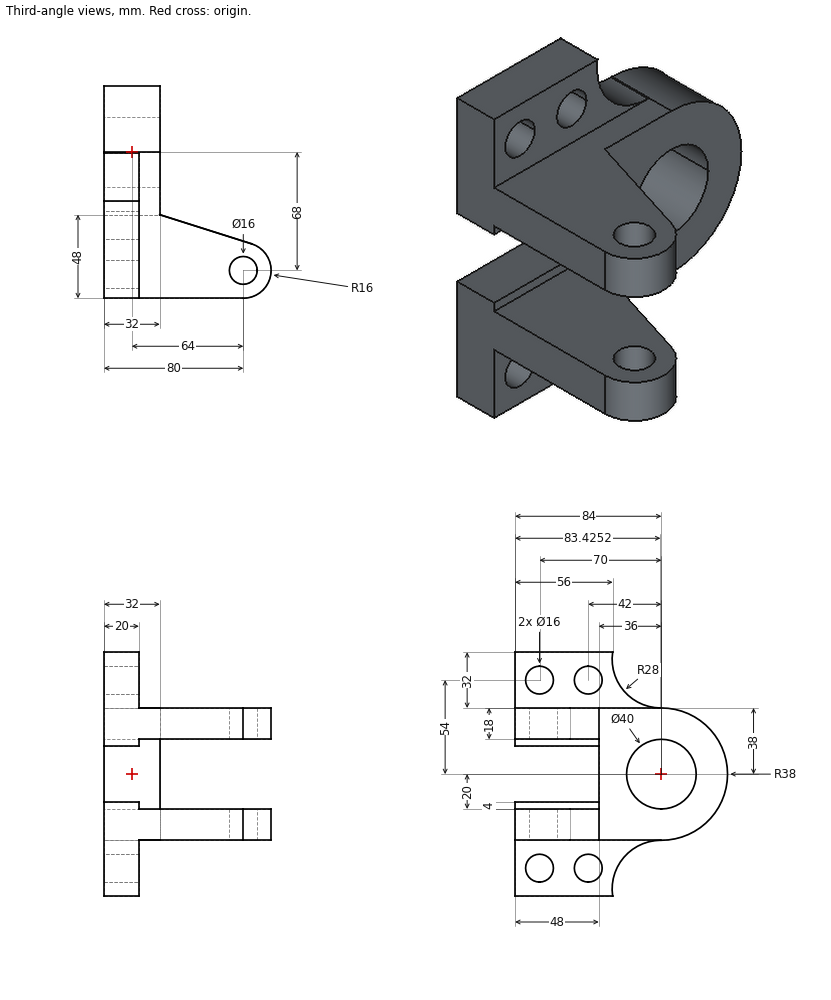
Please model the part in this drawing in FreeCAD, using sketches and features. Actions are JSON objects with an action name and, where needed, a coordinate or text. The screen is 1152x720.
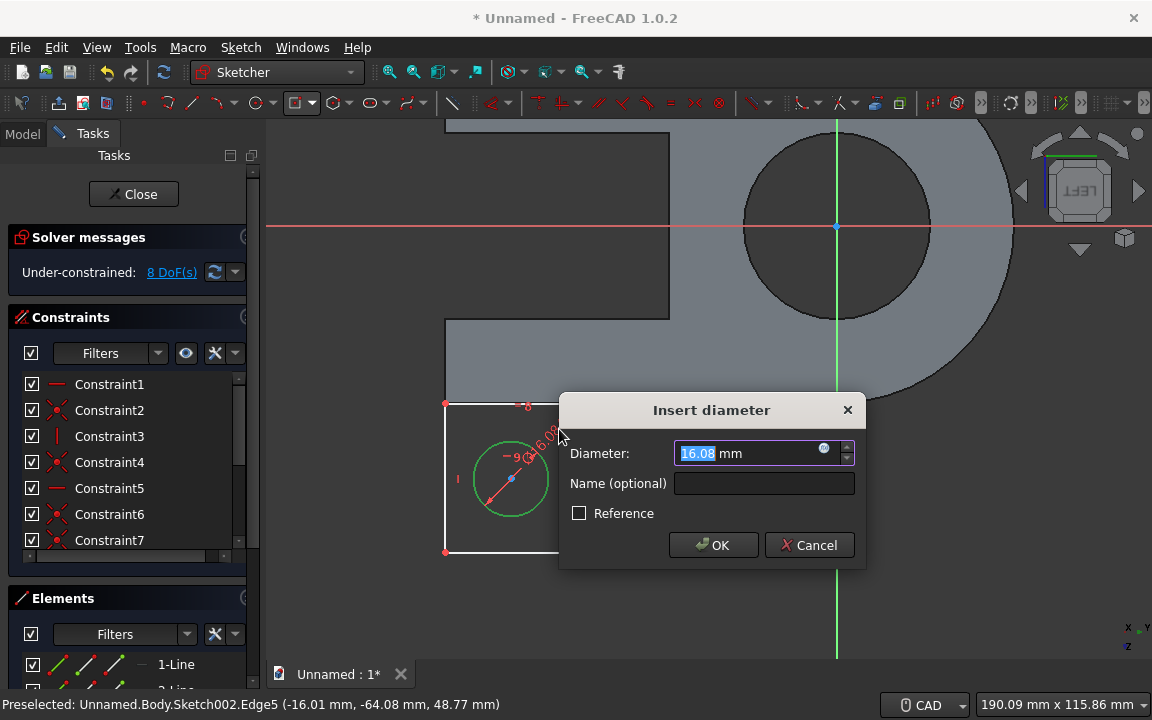
{"action": "type", "text": "16"}
{"action": "key", "text": "Return"}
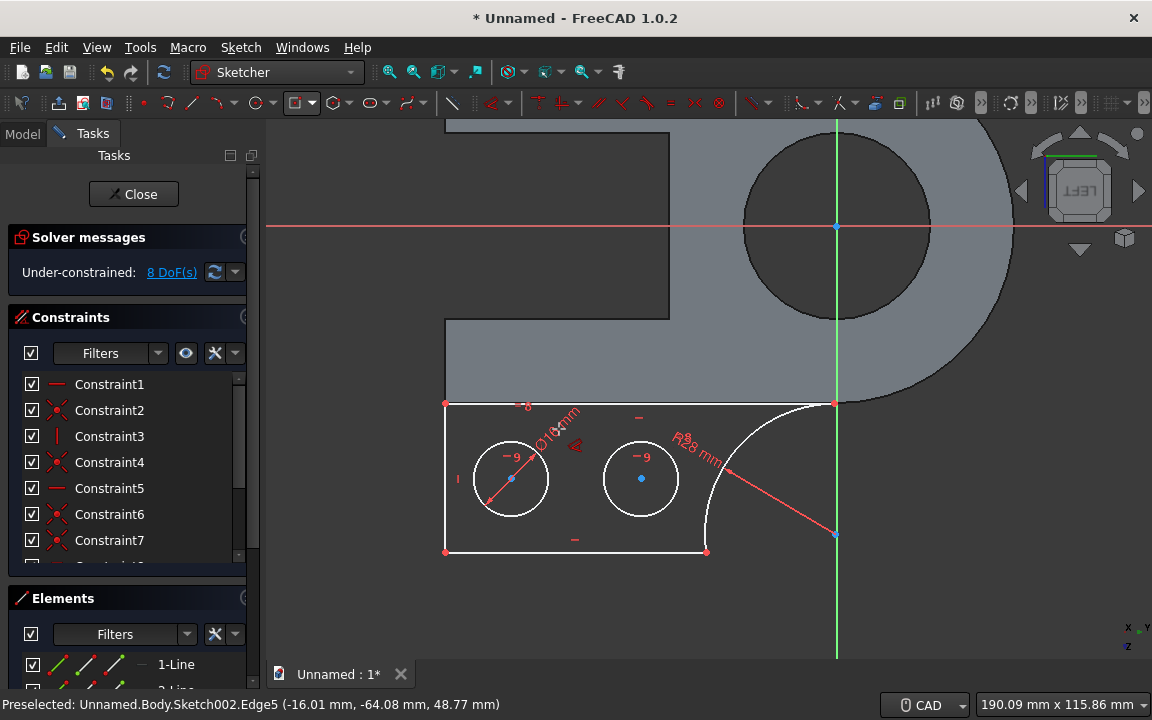
{"action": "left_click", "coordinate": [445, 449]}
{"action": "left_click", "coordinate": [411, 478]}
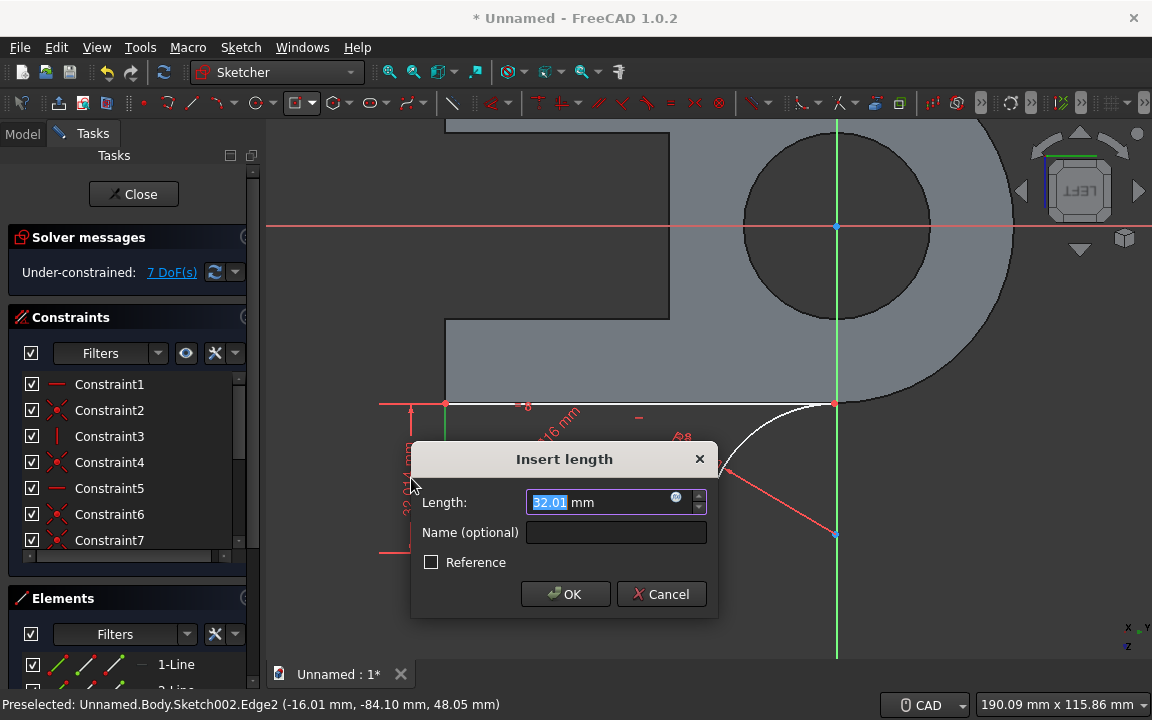
{"action": "type", "text": "32"}
{"action": "key", "text": "Return"}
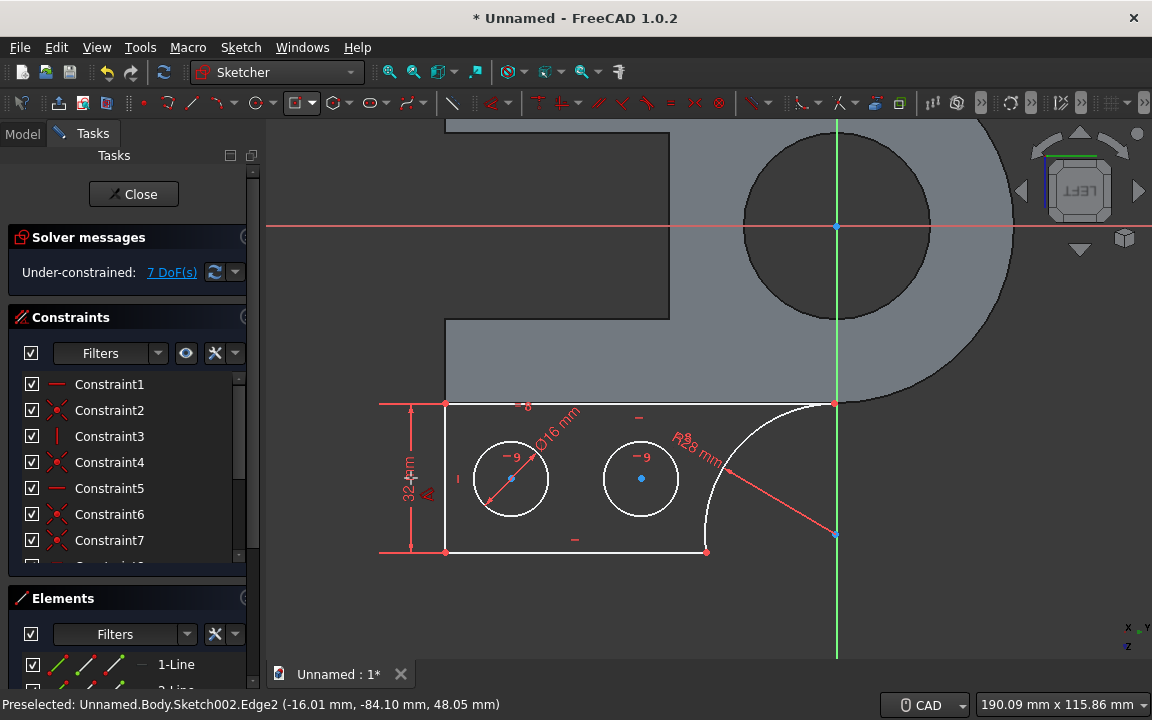
{"action": "left_click", "coordinate": [523, 553]}
{"action": "left_click", "coordinate": [576, 587]}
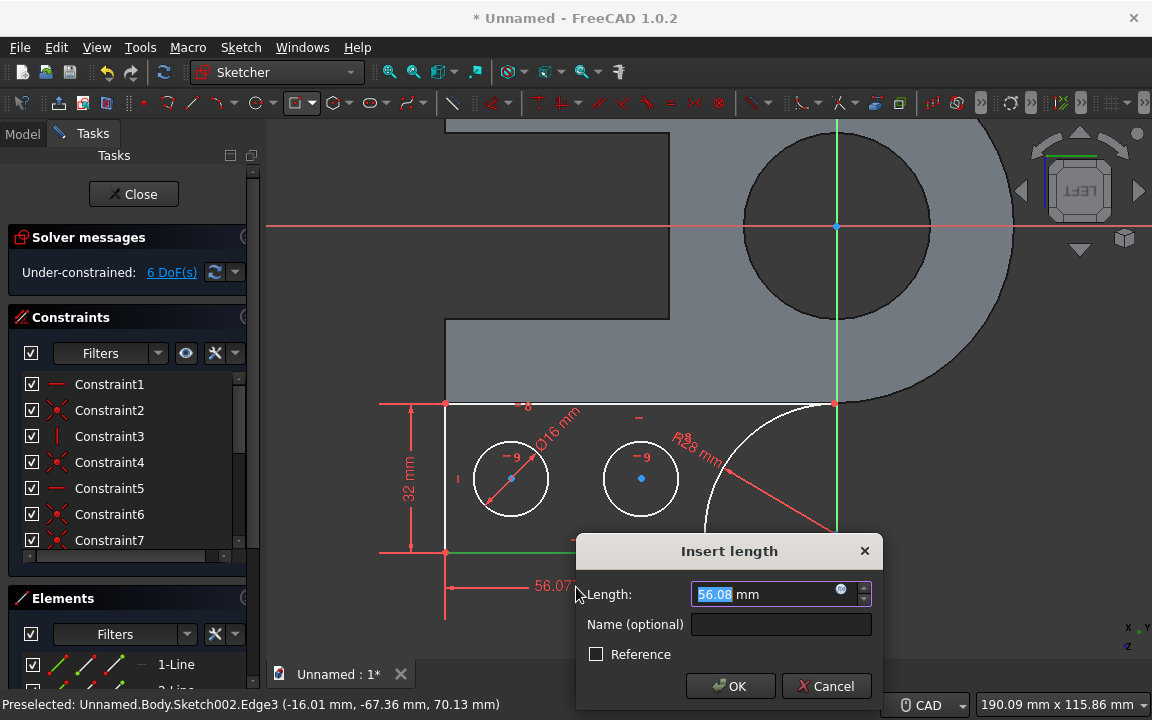
{"action": "type", "text": "56"}
{"action": "key", "text": "Return"}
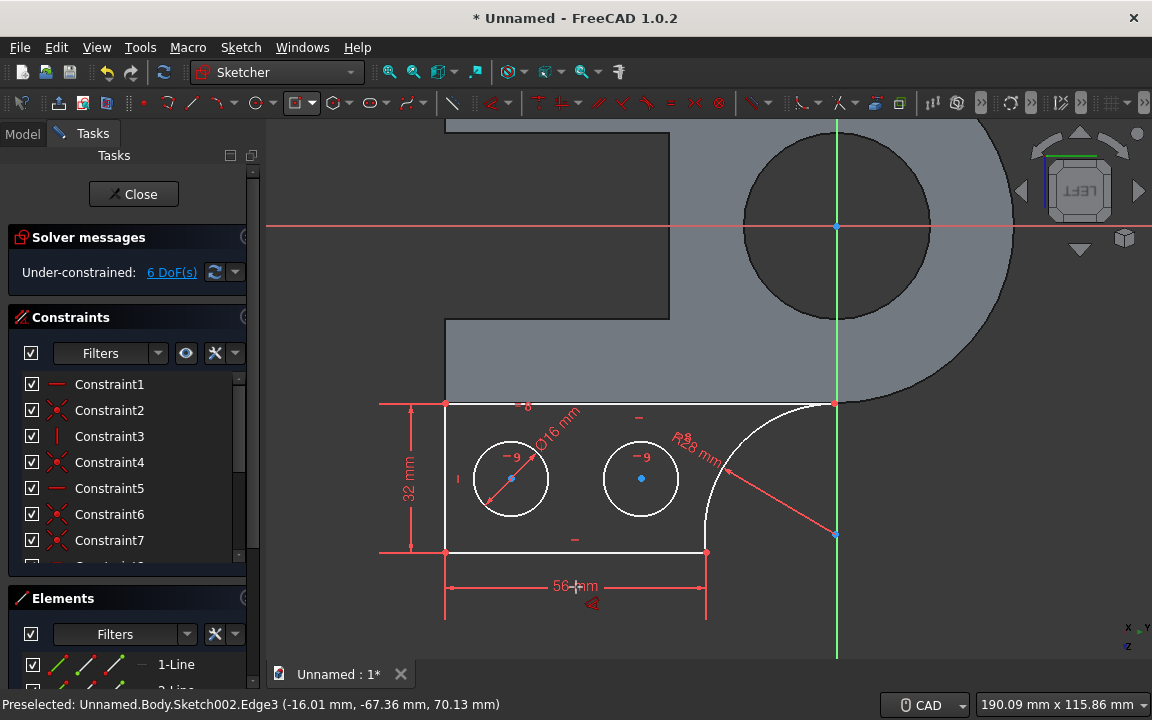
{"action": "left_click", "coordinate": [511, 479]}
{"action": "left_click", "coordinate": [674, 192]}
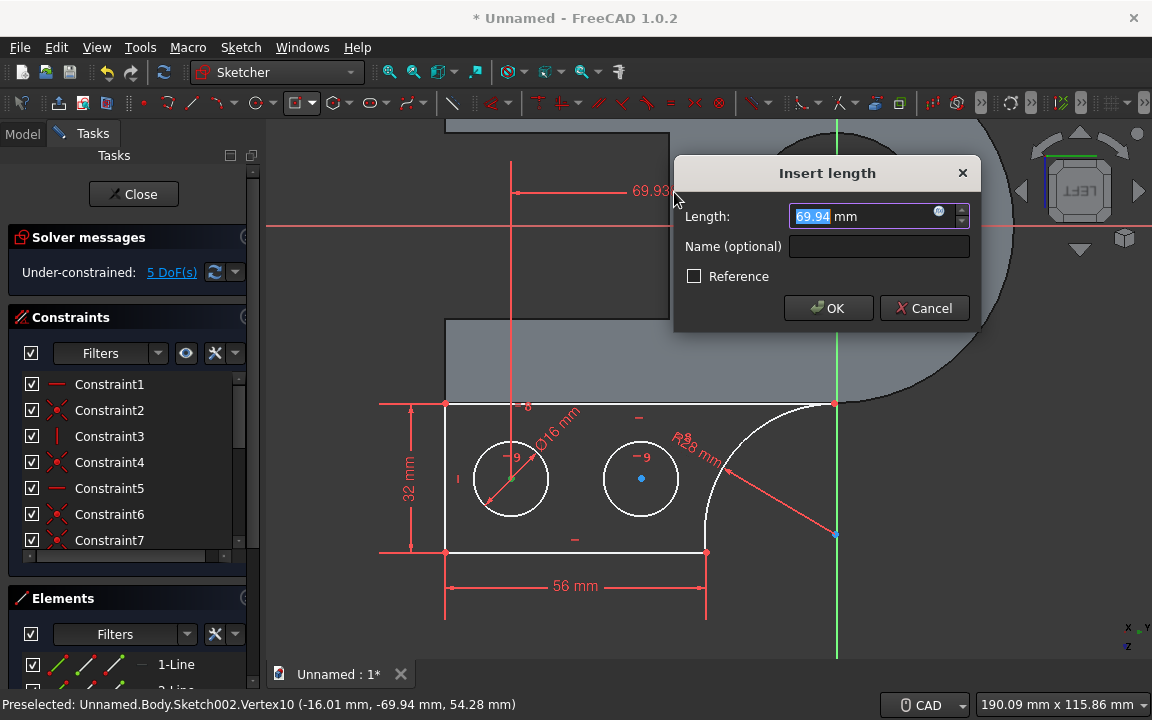
{"action": "type", "text": "70"}
{"action": "key", "text": "Return"}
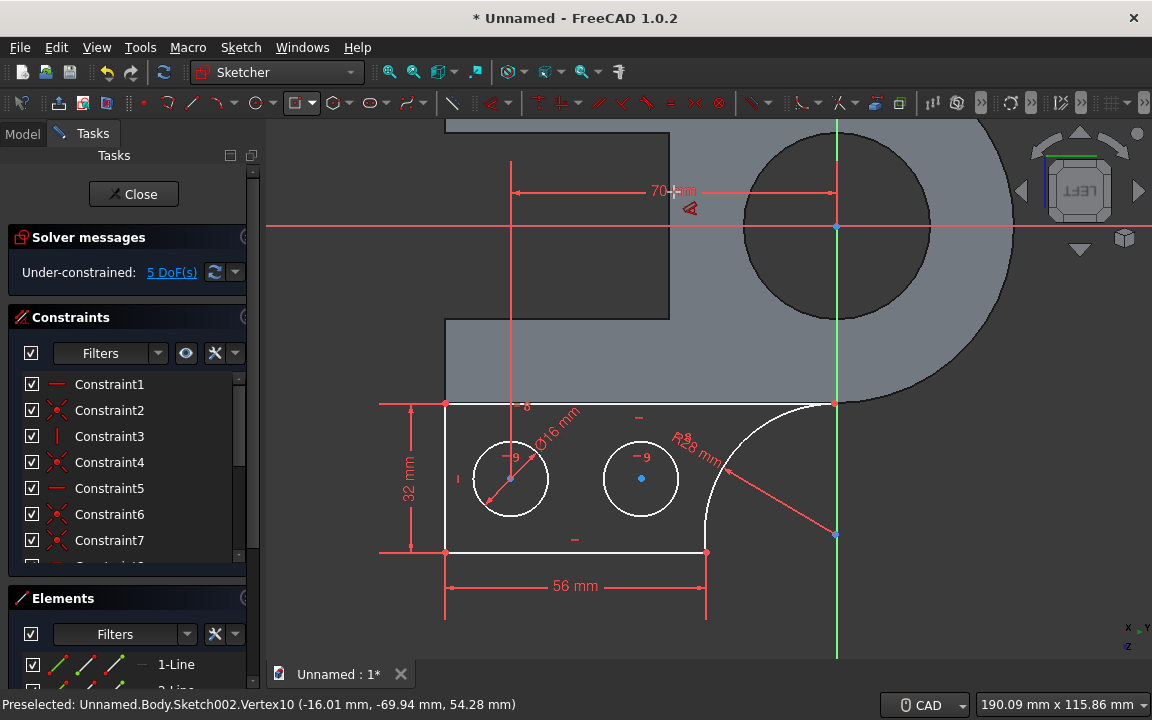
{"action": "left_click", "coordinate": [511, 479]}
{"action": "left_click", "coordinate": [871, 353]}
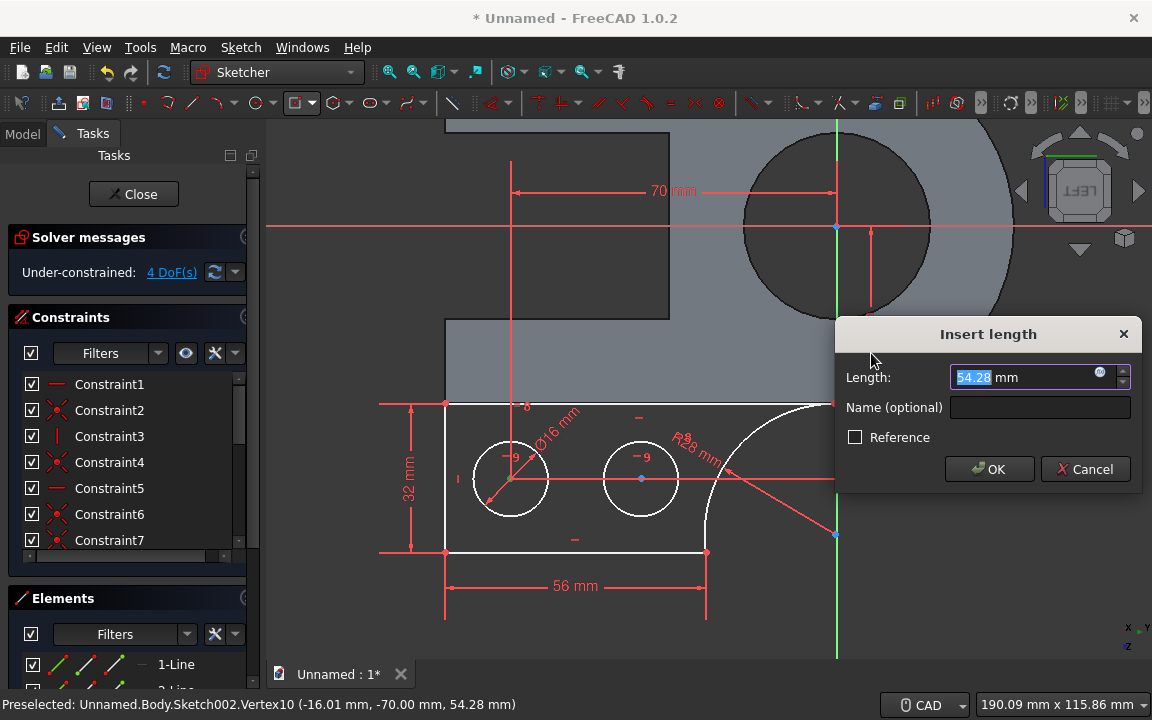
{"action": "type", "text": "54"}
{"action": "key", "text": "Return"}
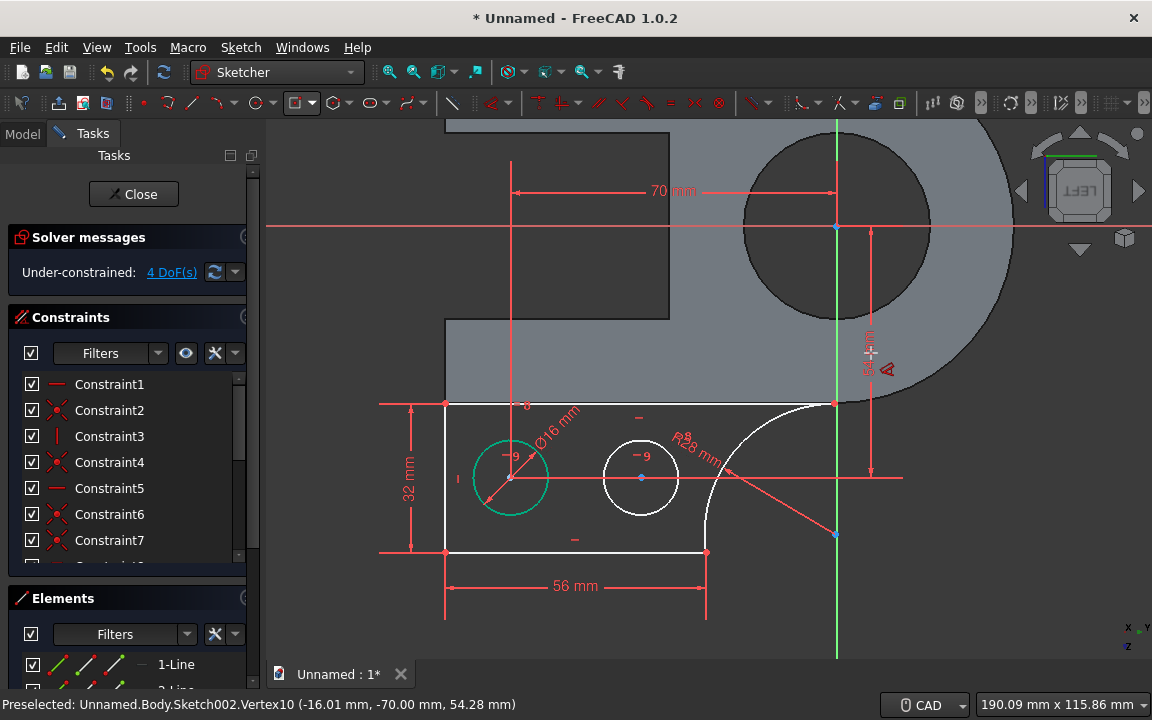
{"action": "left_click", "coordinate": [641, 478]}
{"action": "left_click", "coordinate": [784, 192]}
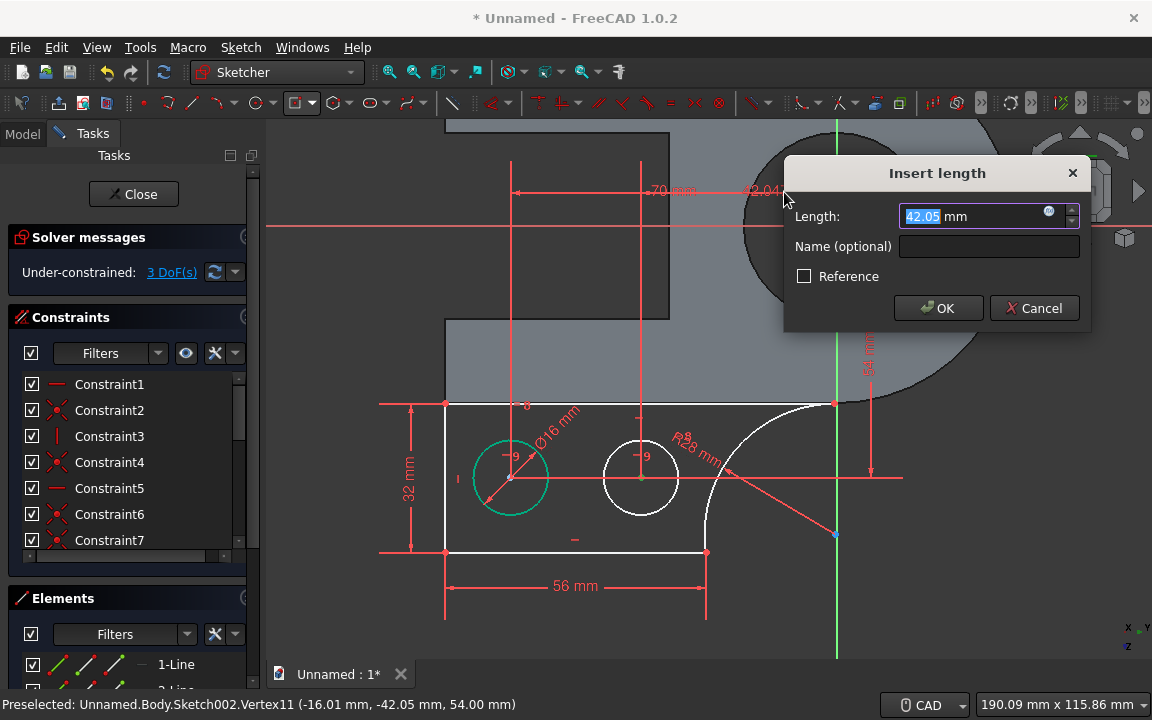
{"action": "type", "text": "42"}
{"action": "key", "text": "Return"}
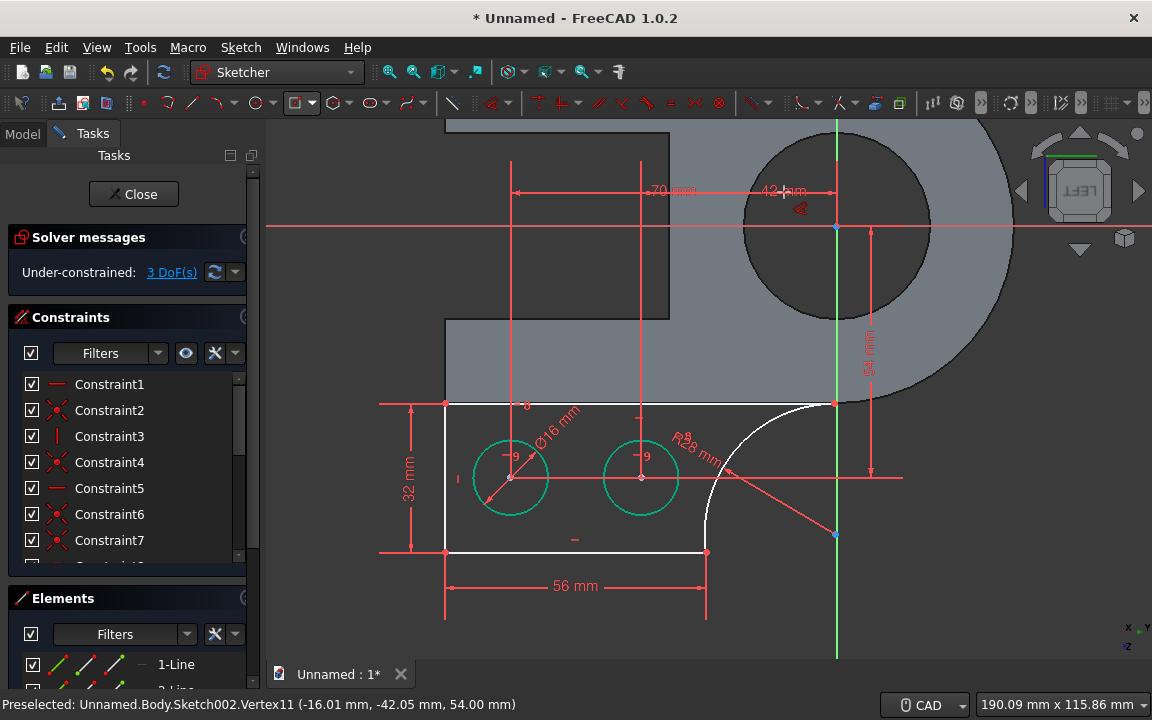
{"action": "left_click", "coordinate": [834, 404]}
{"action": "left_click", "coordinate": [871, 315]}